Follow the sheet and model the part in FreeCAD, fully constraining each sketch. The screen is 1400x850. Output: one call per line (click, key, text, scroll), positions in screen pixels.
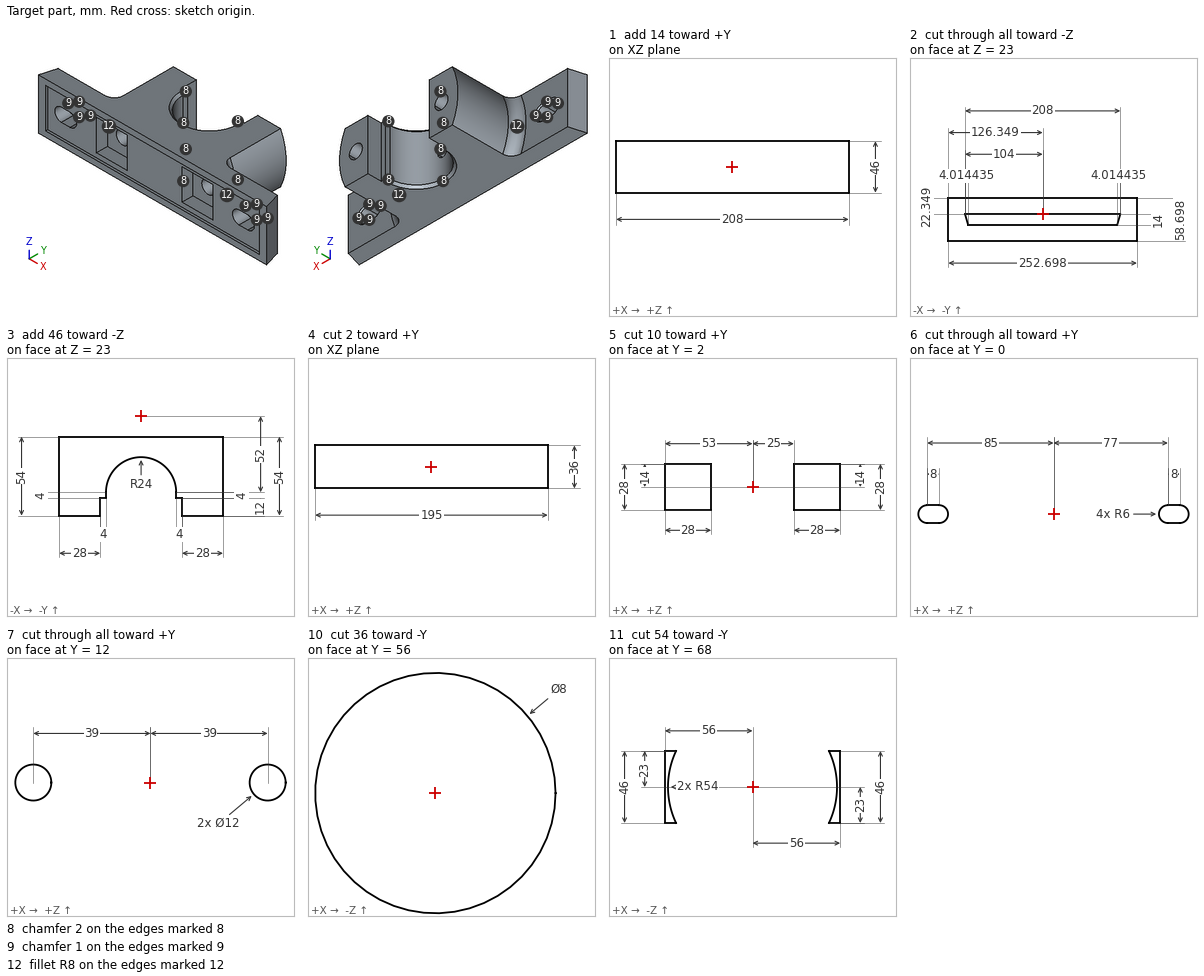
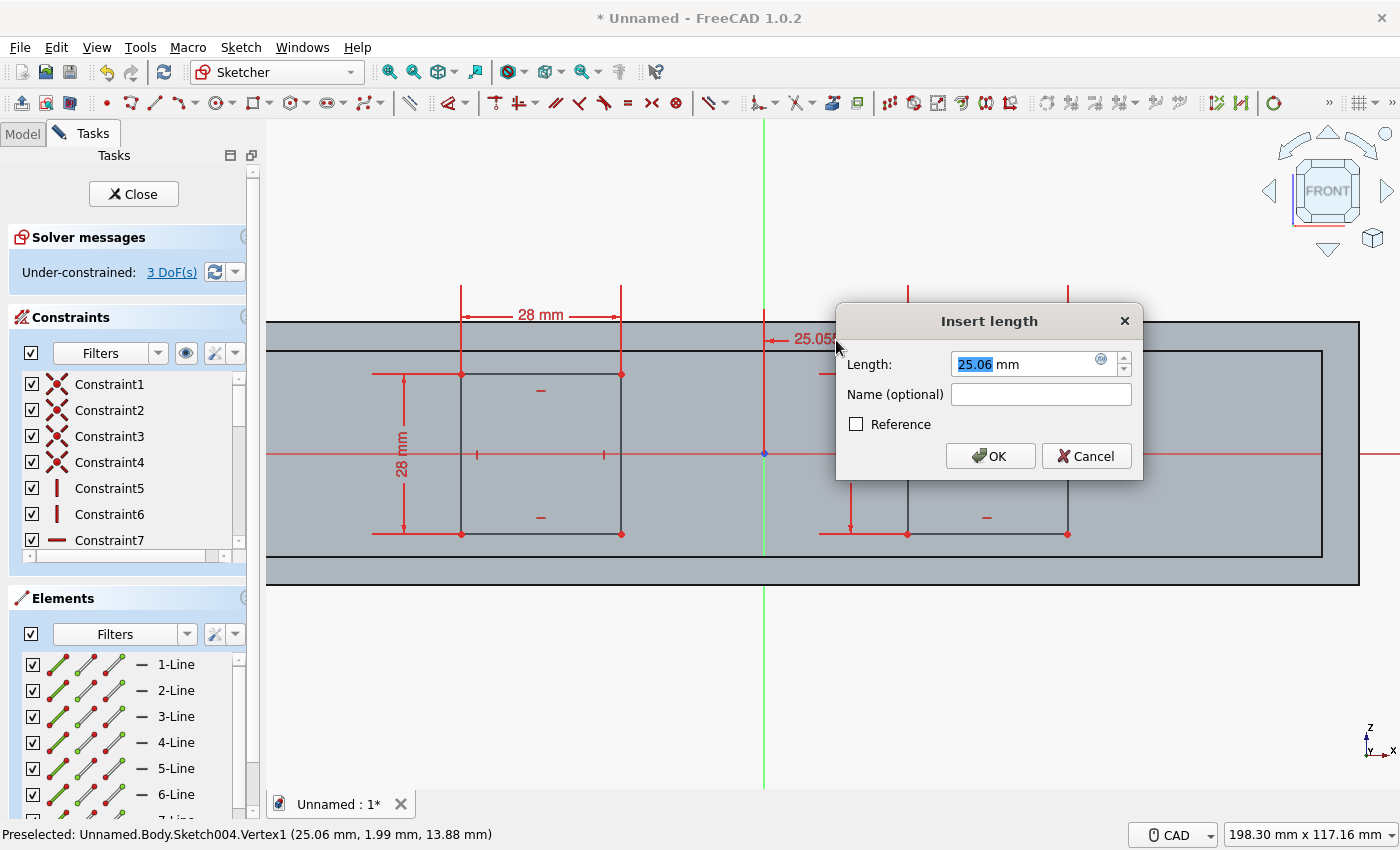
text(25)
key(Return)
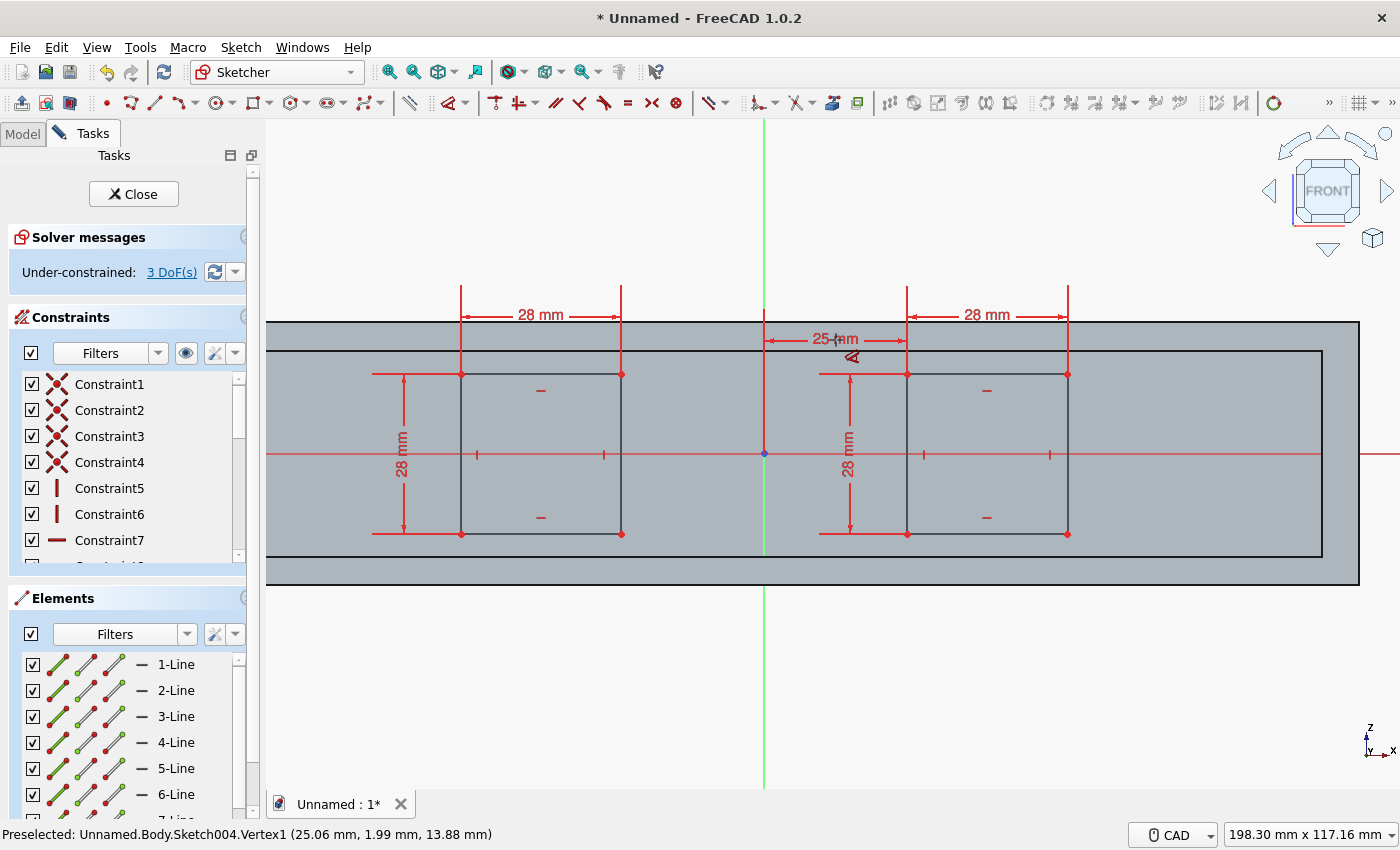
click(907, 374)
click(941, 414)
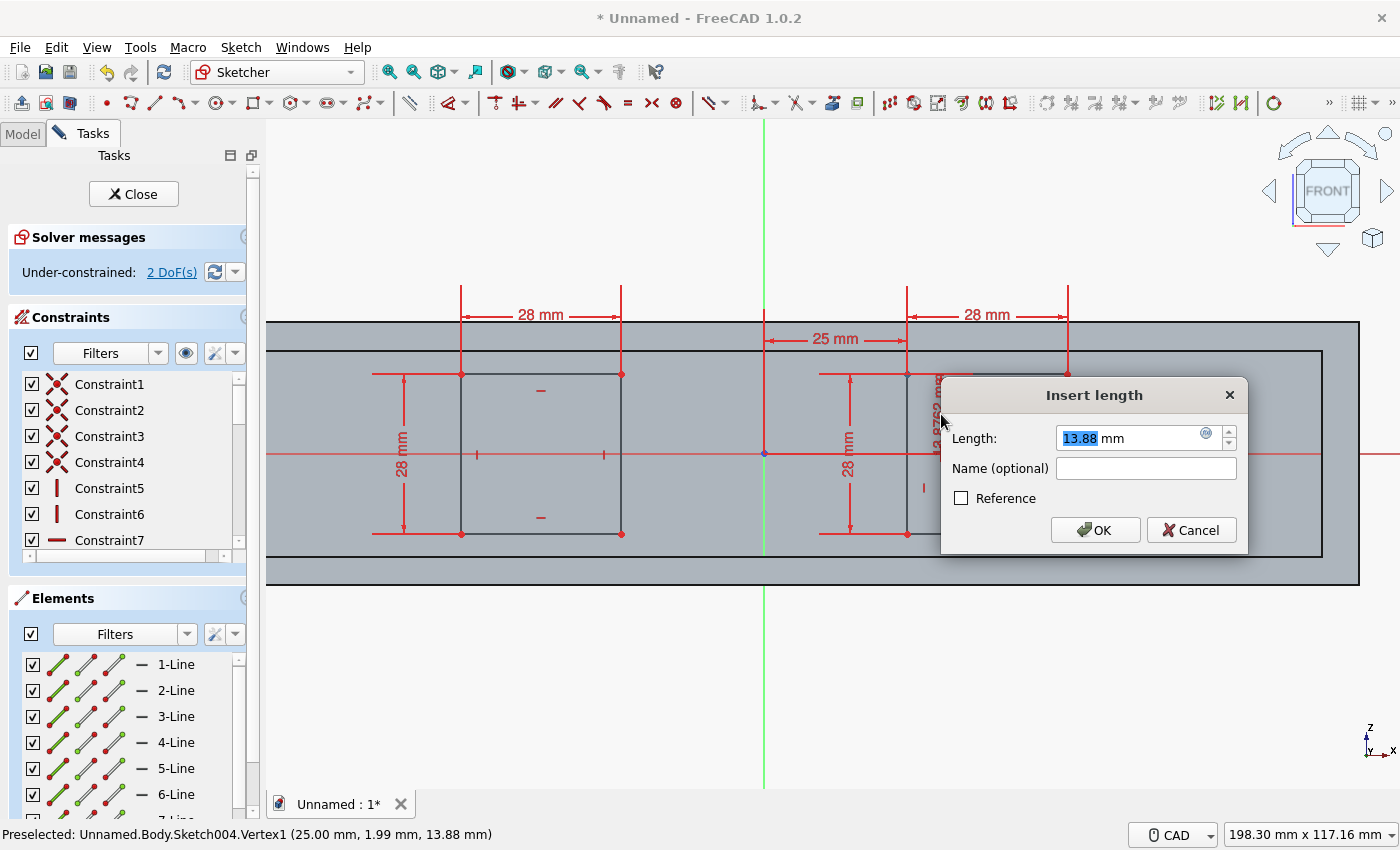
text(14)
key(Return)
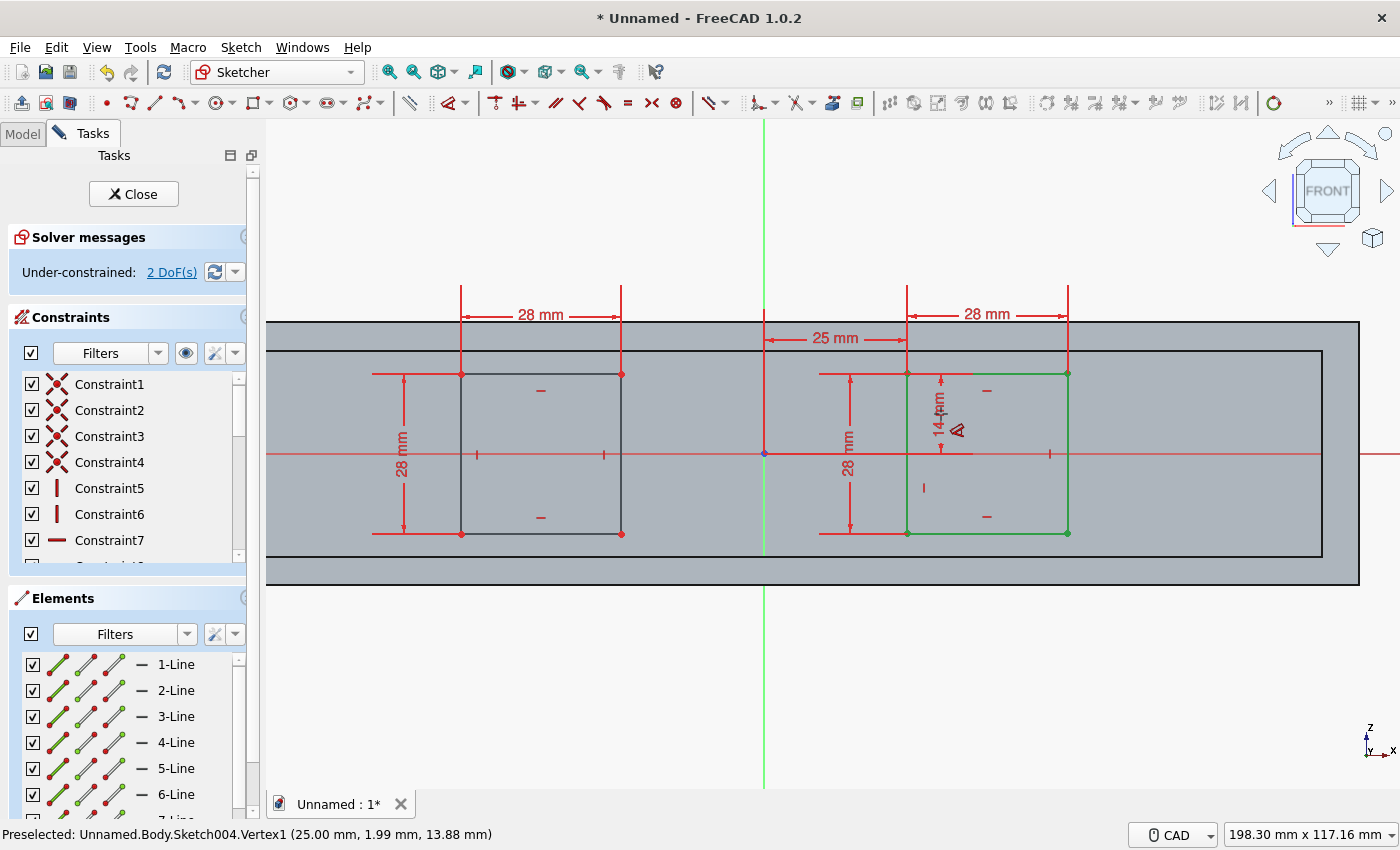
click(461, 374)
click(613, 340)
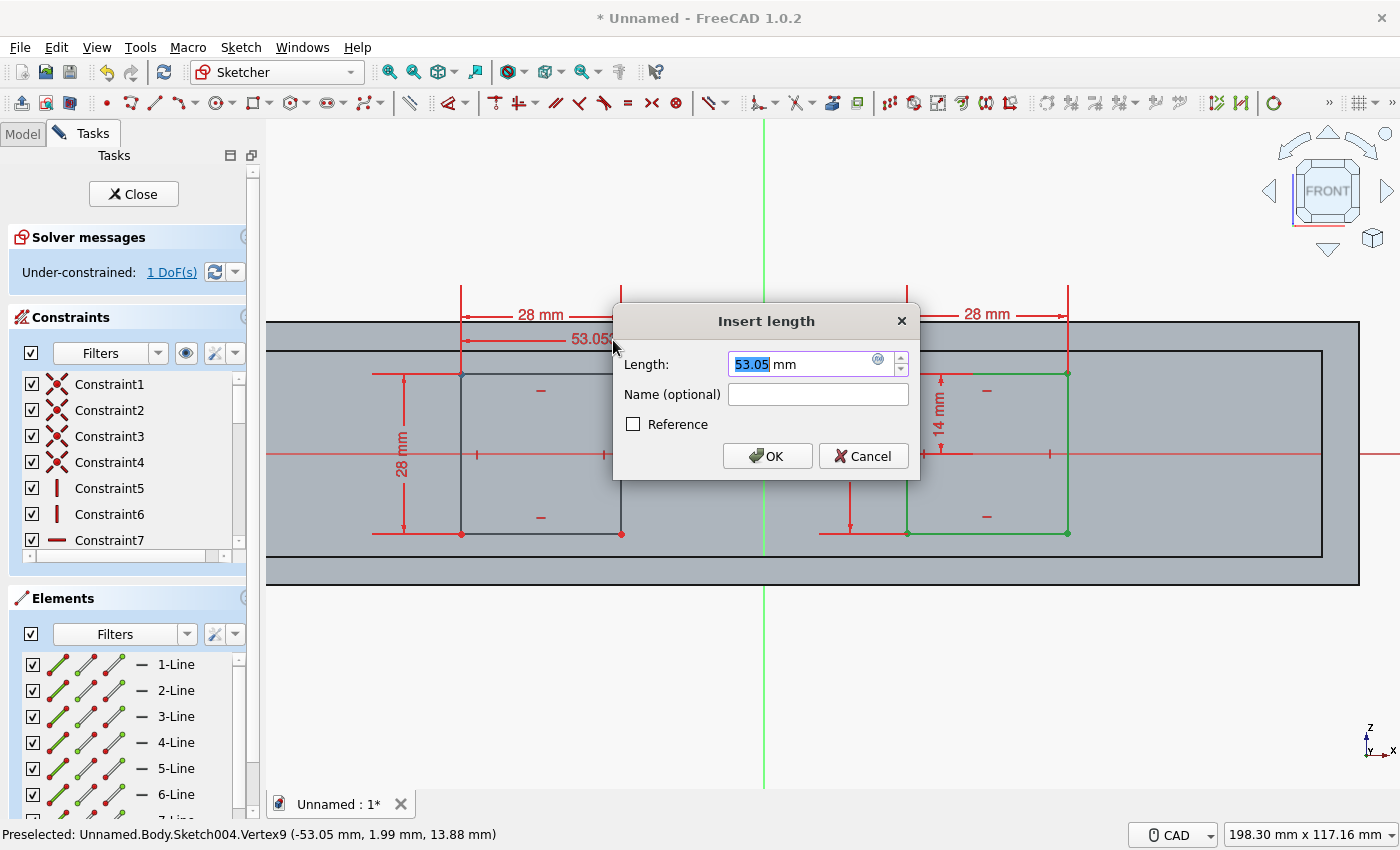
text(53)
key(Return)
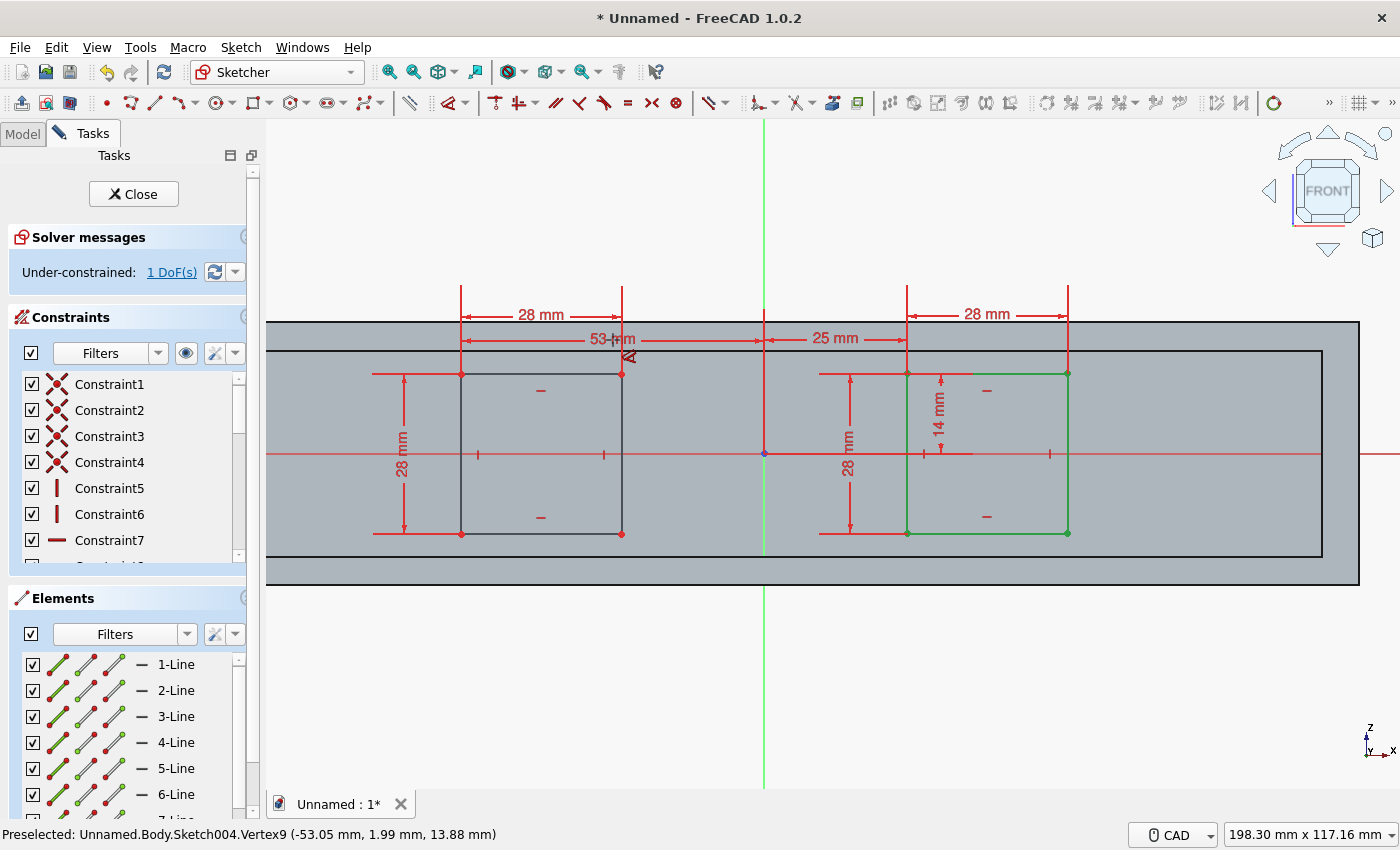
click(461, 374)
click(427, 414)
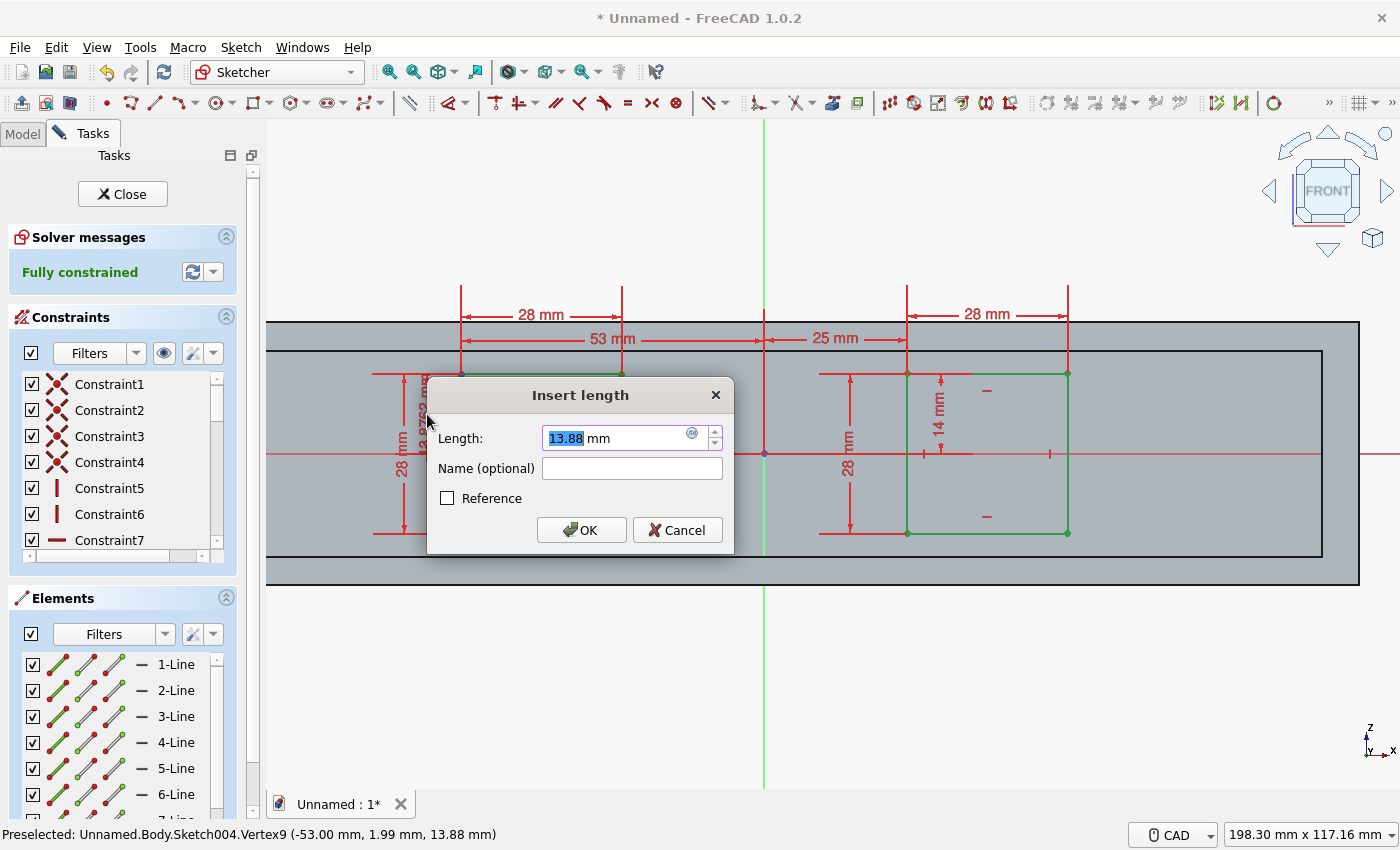
text(14)
key(Return)
key(Escape)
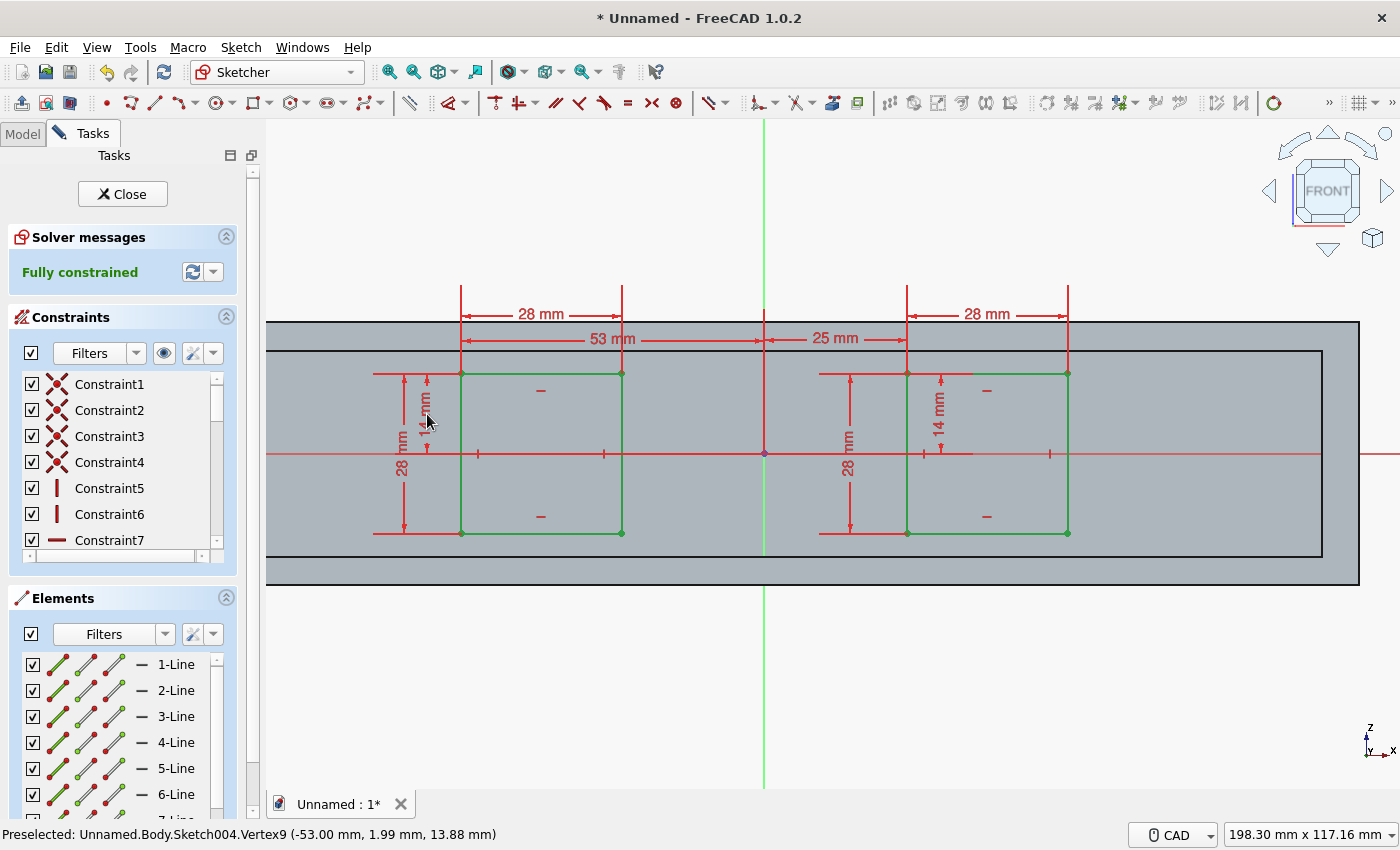
click(123, 194)